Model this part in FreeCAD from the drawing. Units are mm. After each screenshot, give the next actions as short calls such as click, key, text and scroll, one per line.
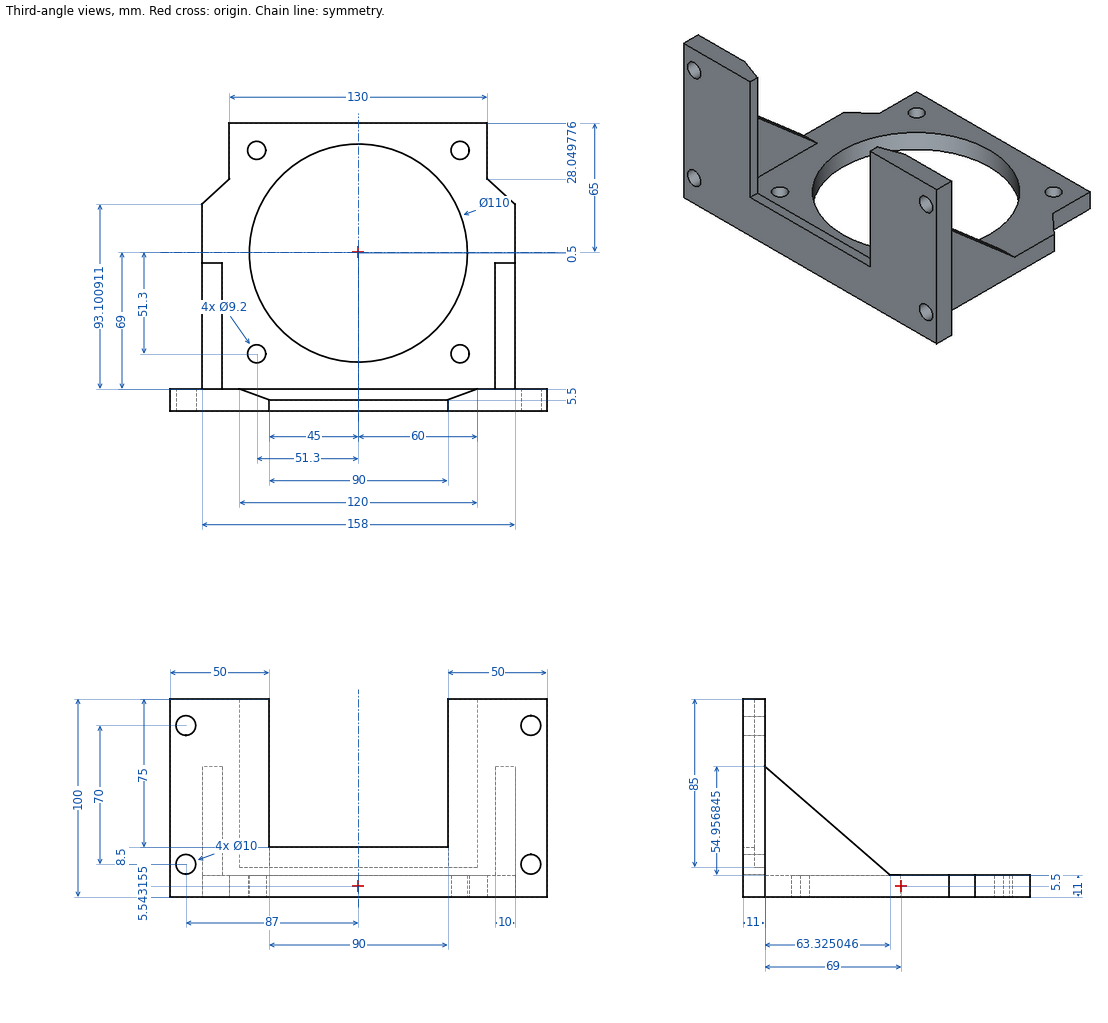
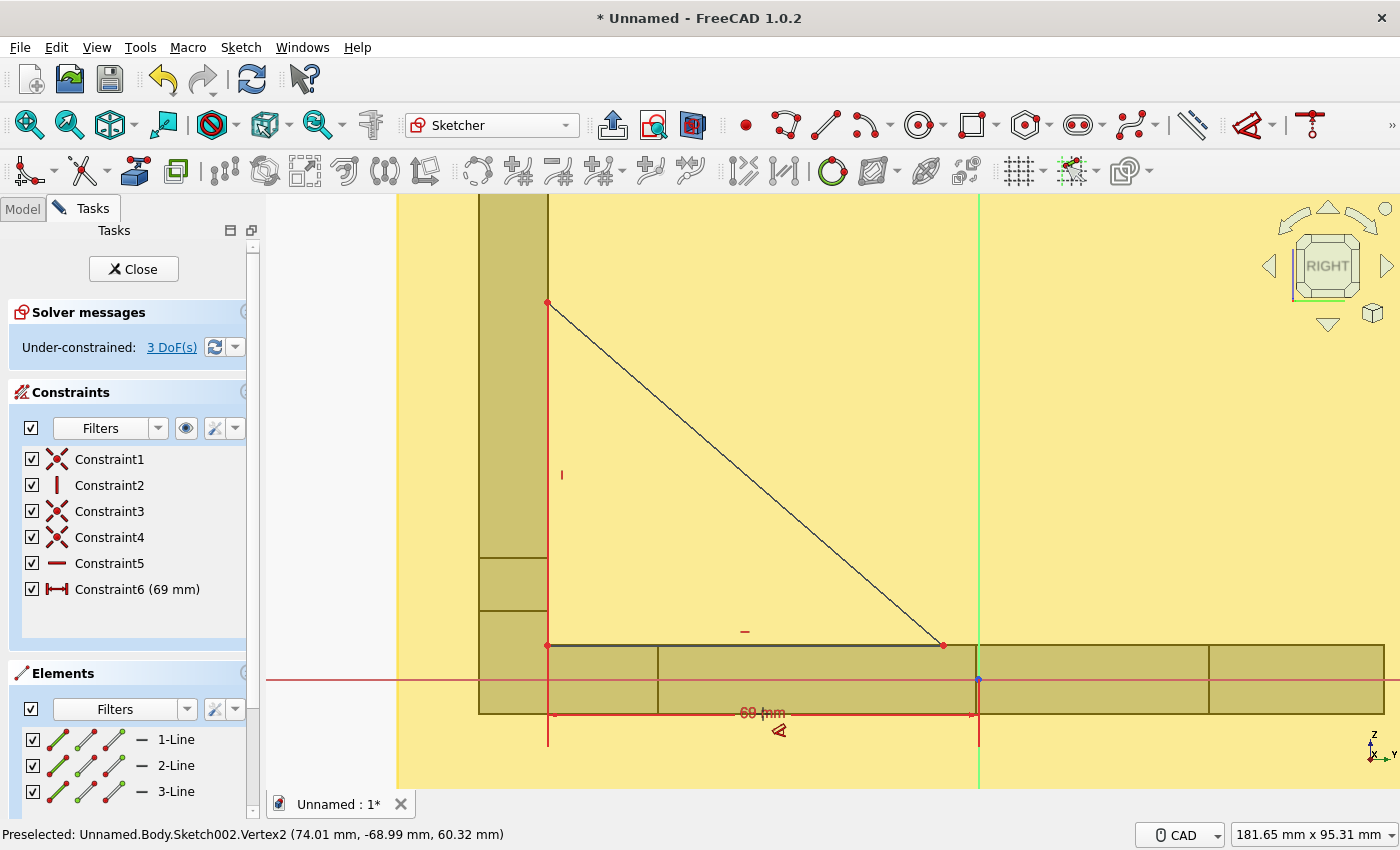
click(943, 646)
click(1013, 663)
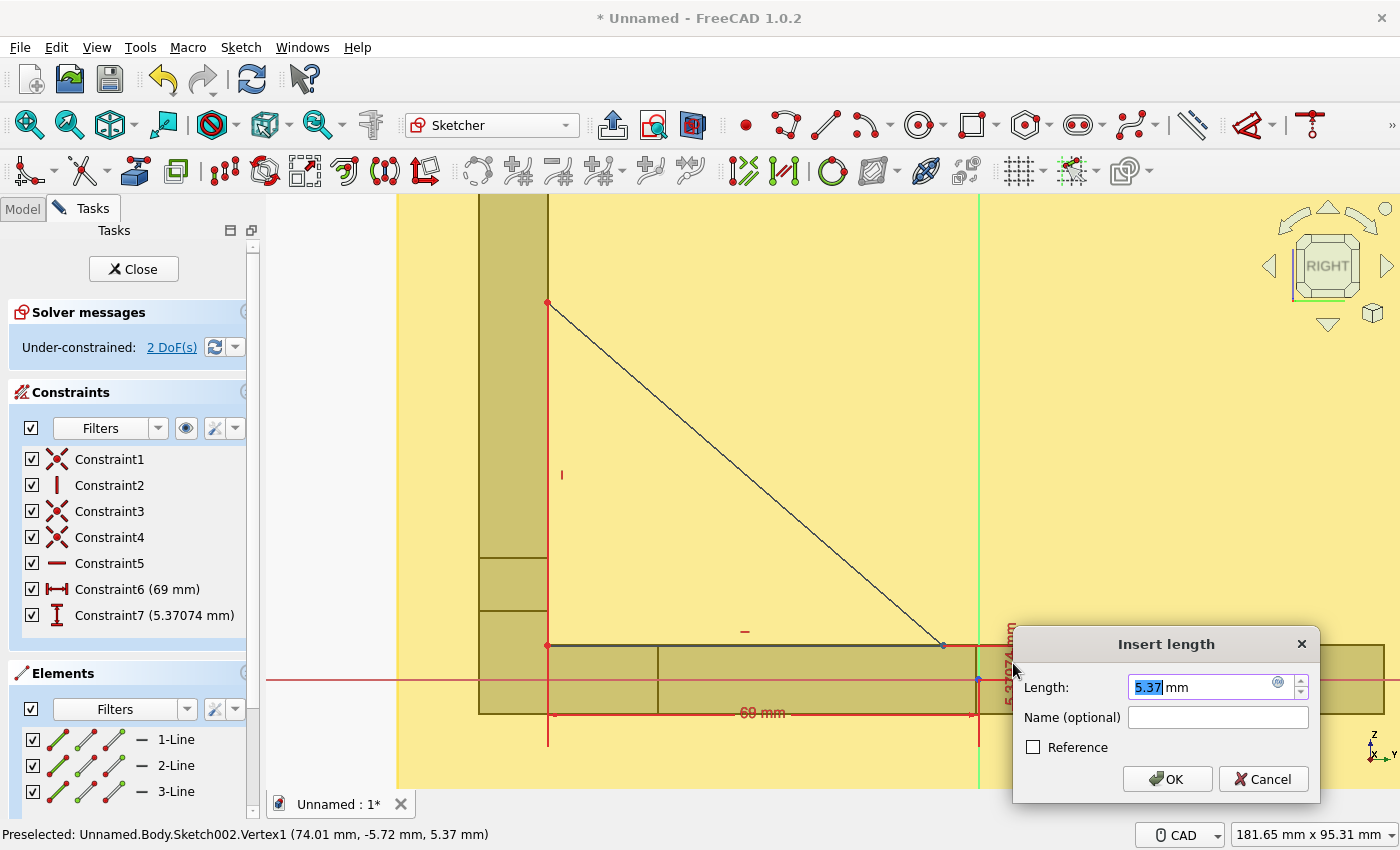
text(5.5)
key(Return)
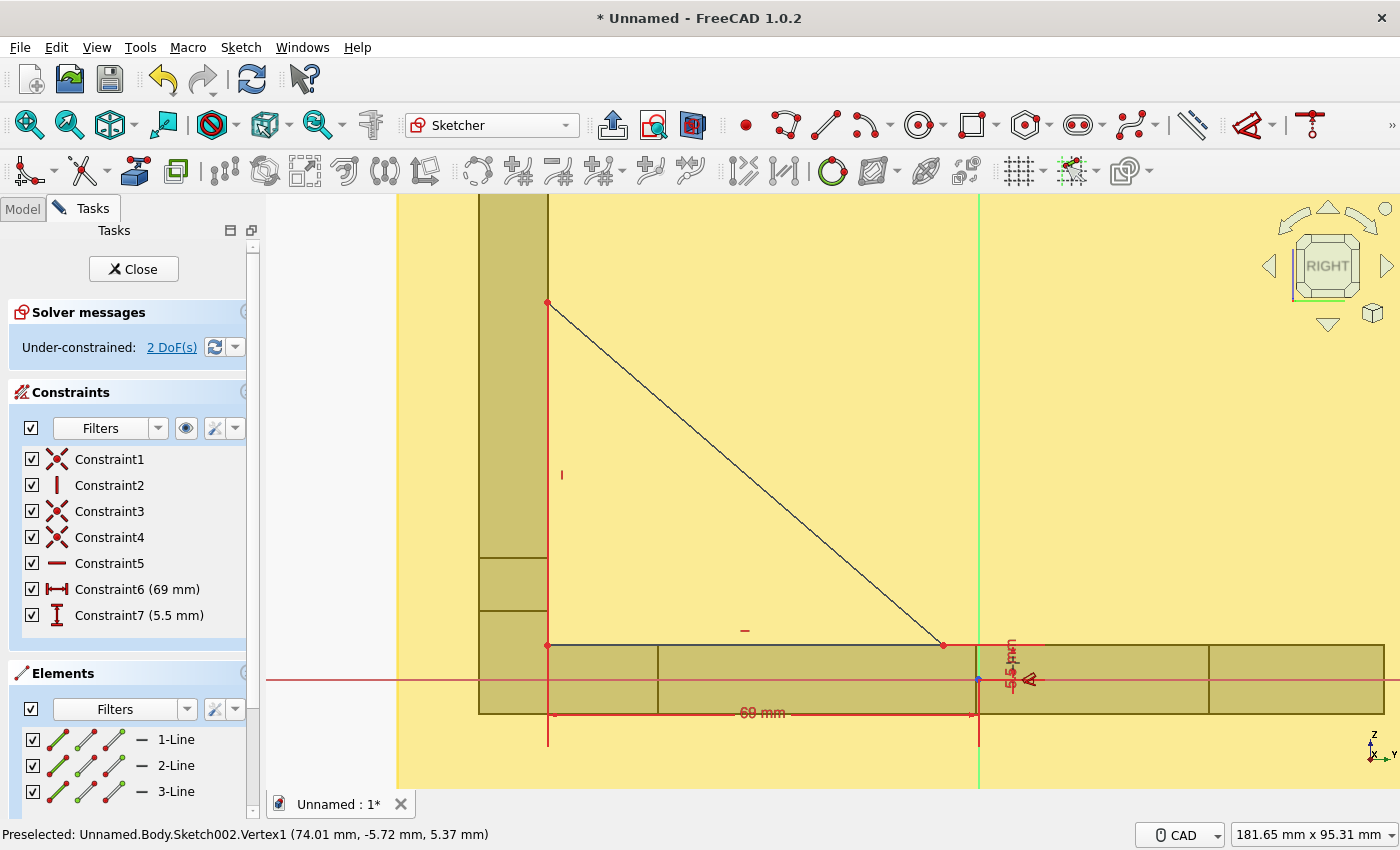
click(548, 406)
click(514, 474)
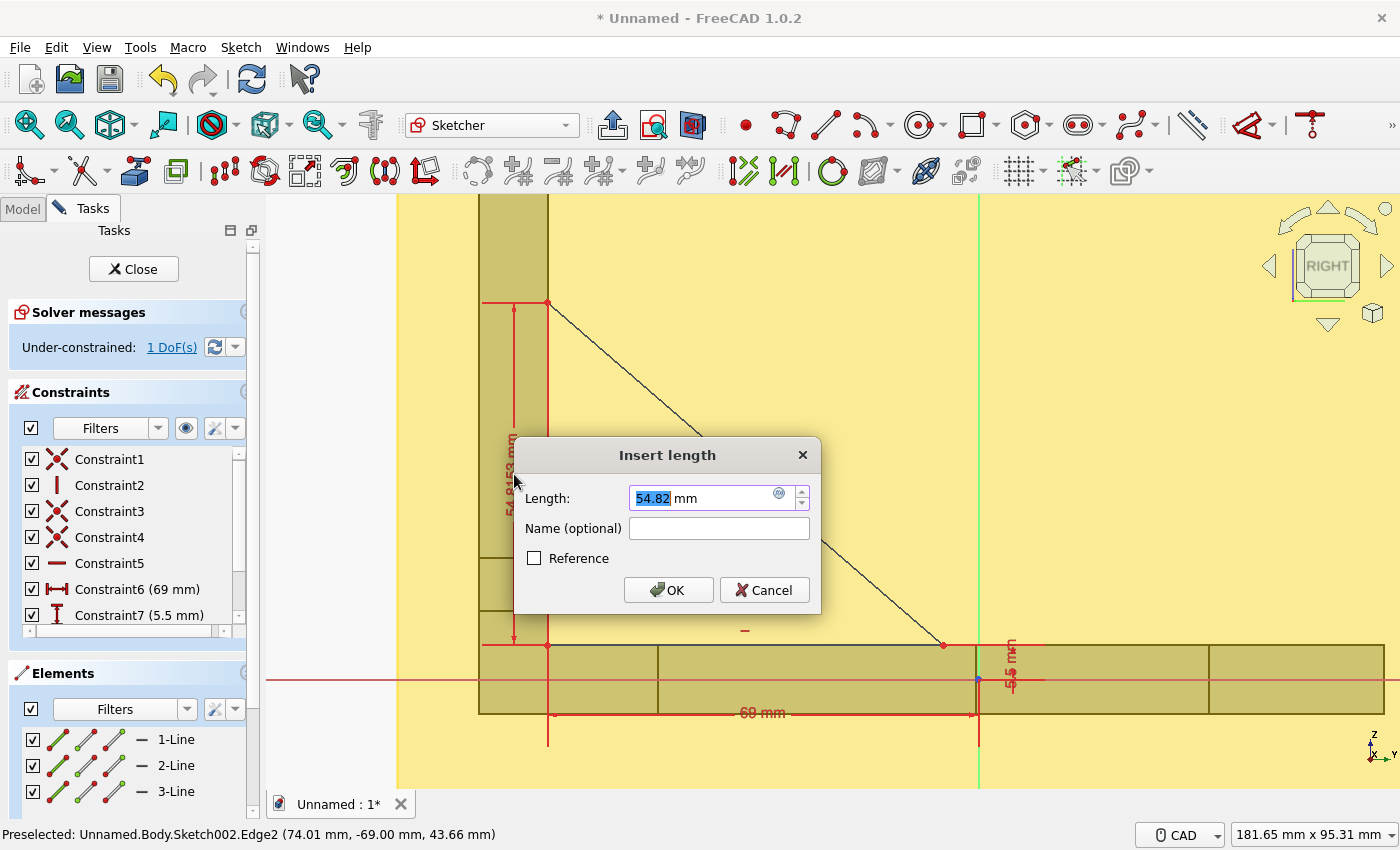
text(54.956845)
key(Return)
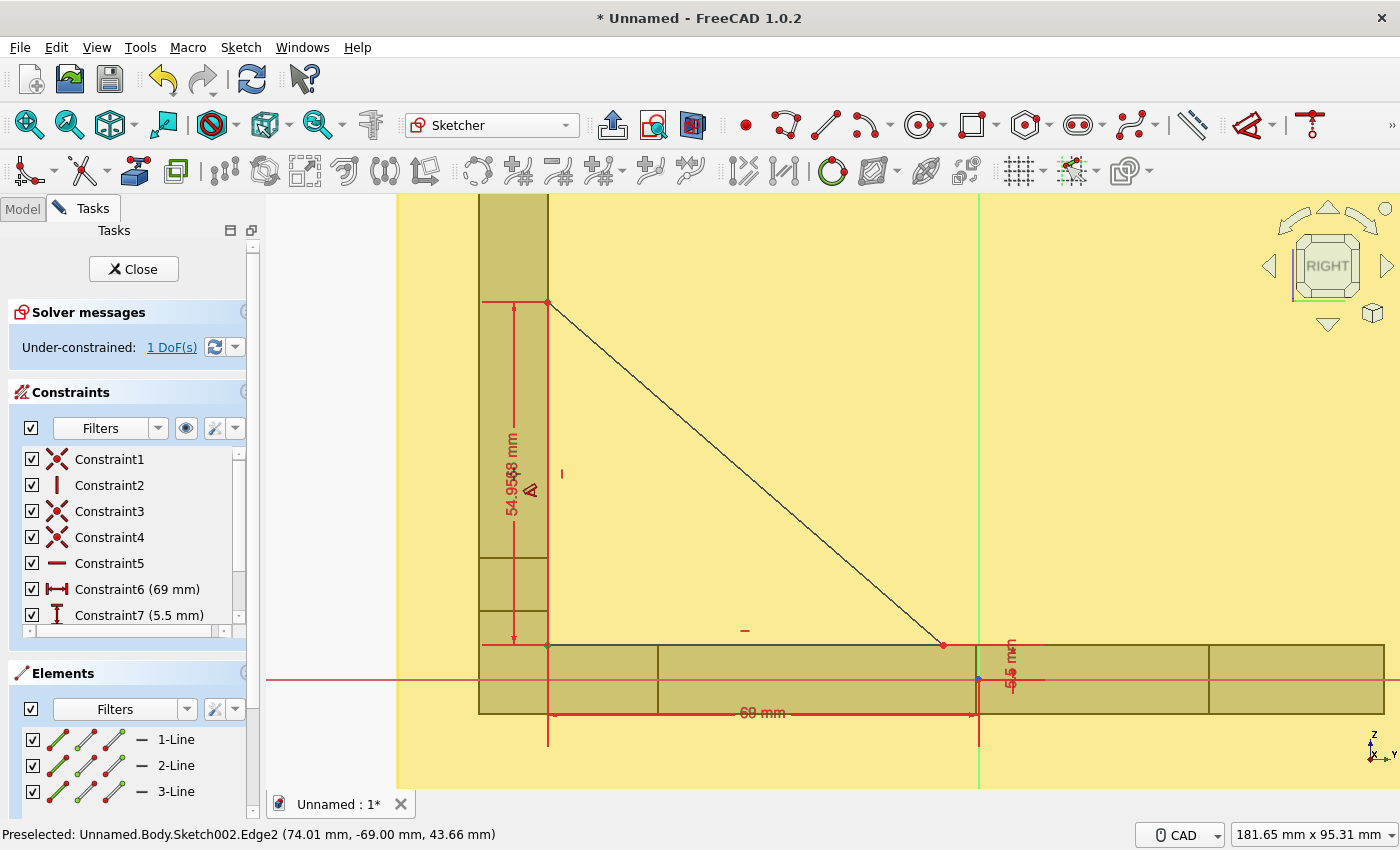
click(666, 645)
click(745, 611)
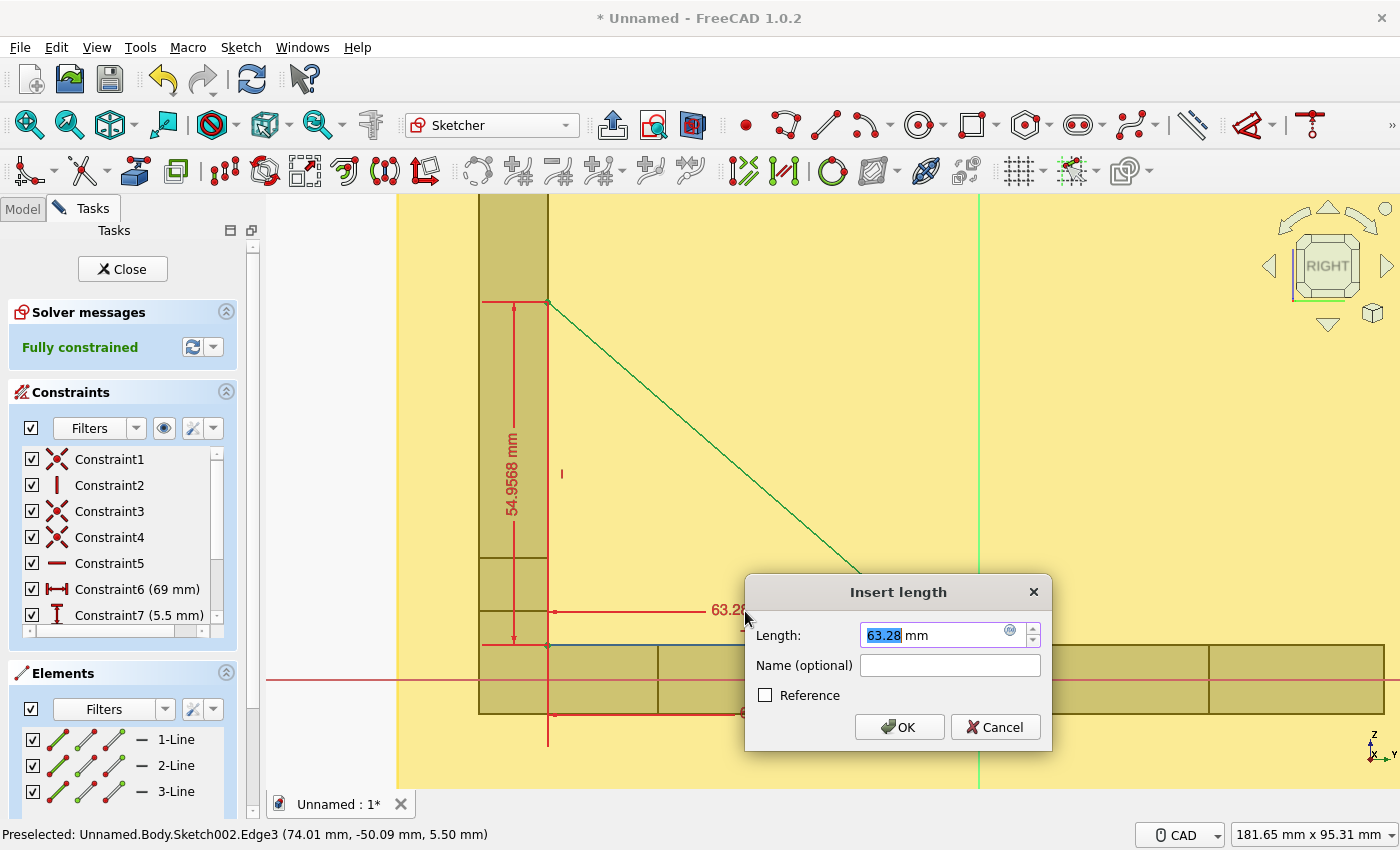
text(63.325046)
key(Return)
key(Escape)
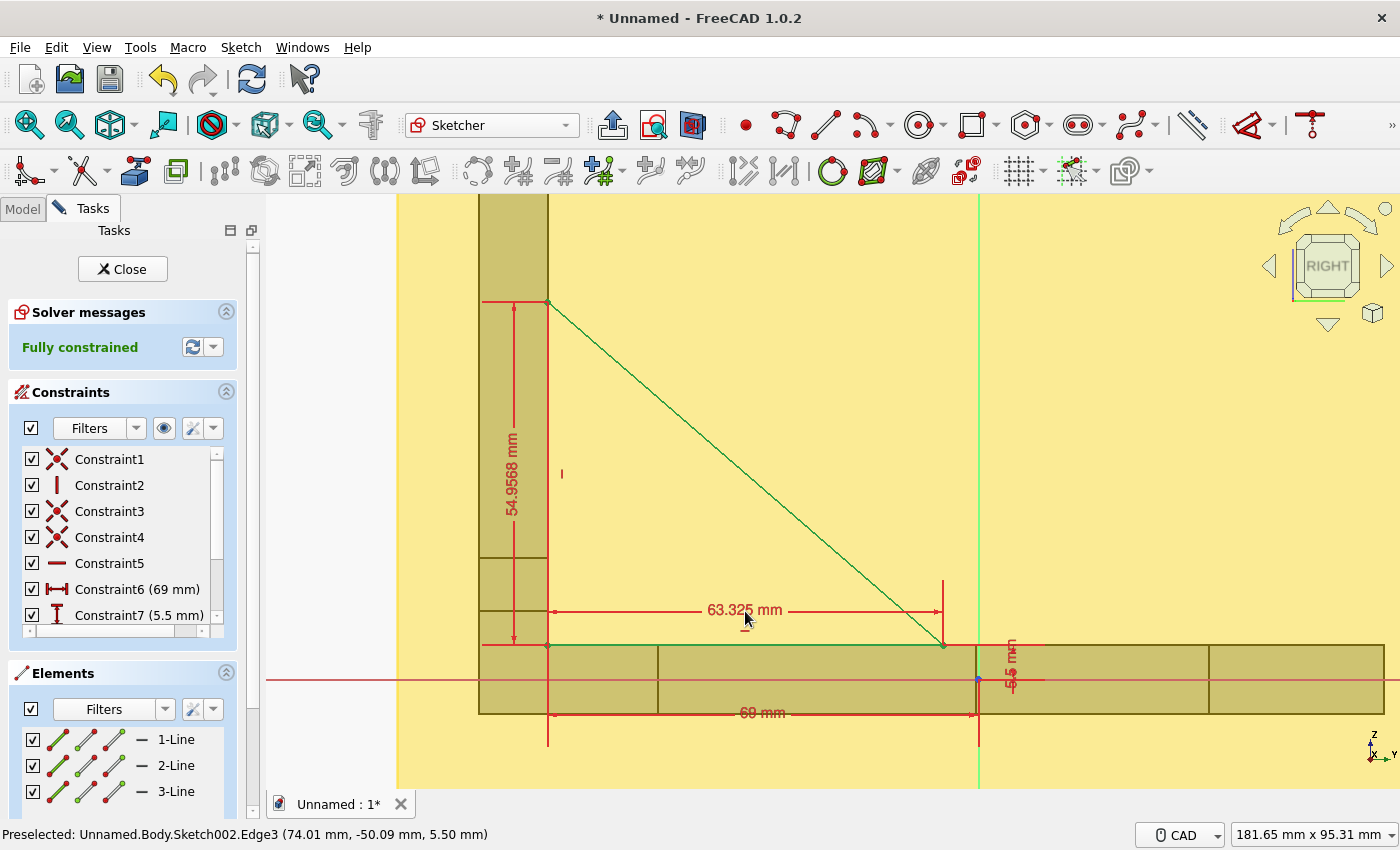
click(123, 269)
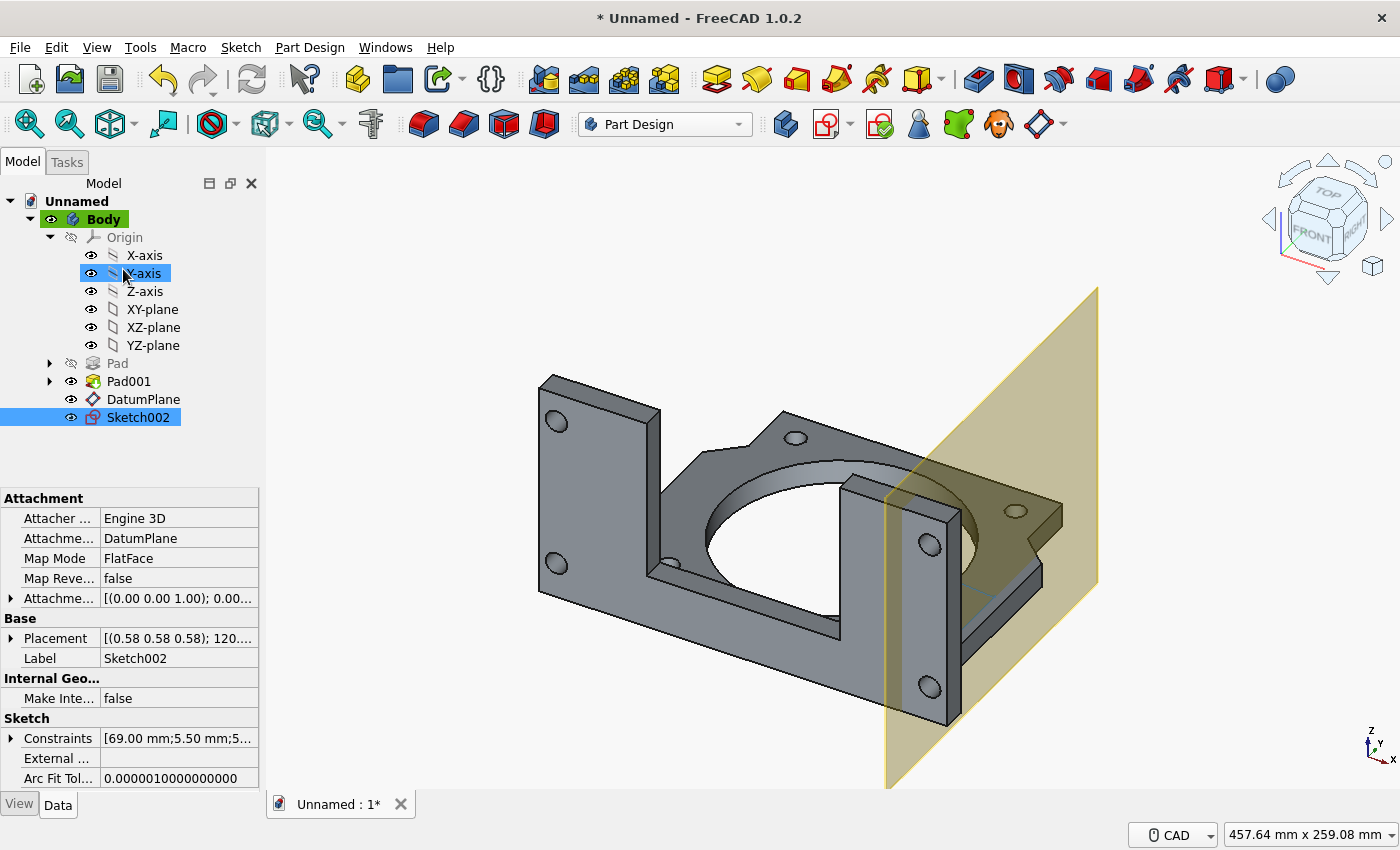
click(718, 80)